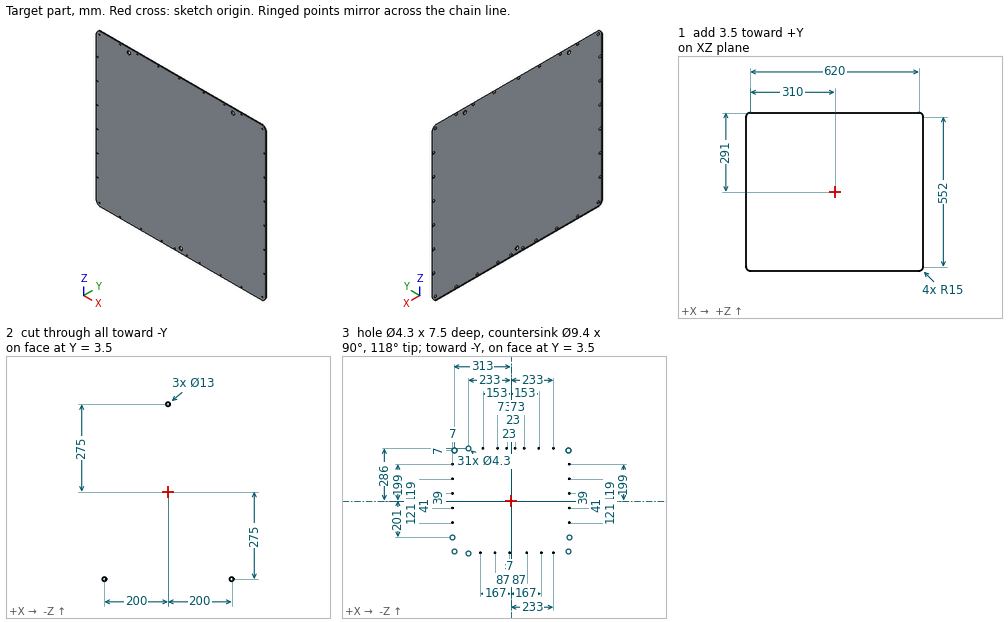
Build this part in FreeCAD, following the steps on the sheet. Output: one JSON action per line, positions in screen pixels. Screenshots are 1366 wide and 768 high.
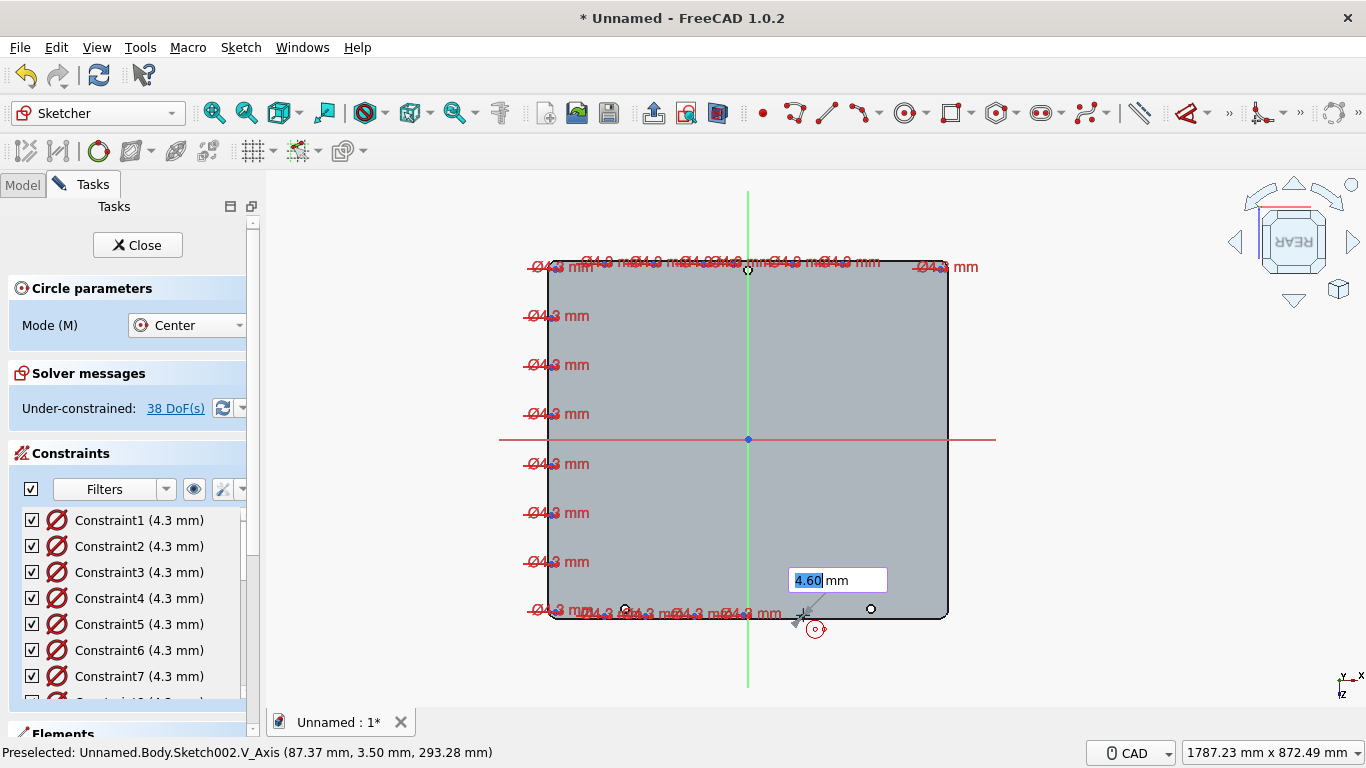
{"action": "type", "text": "4.3"}
{"action": "key", "text": "Return"}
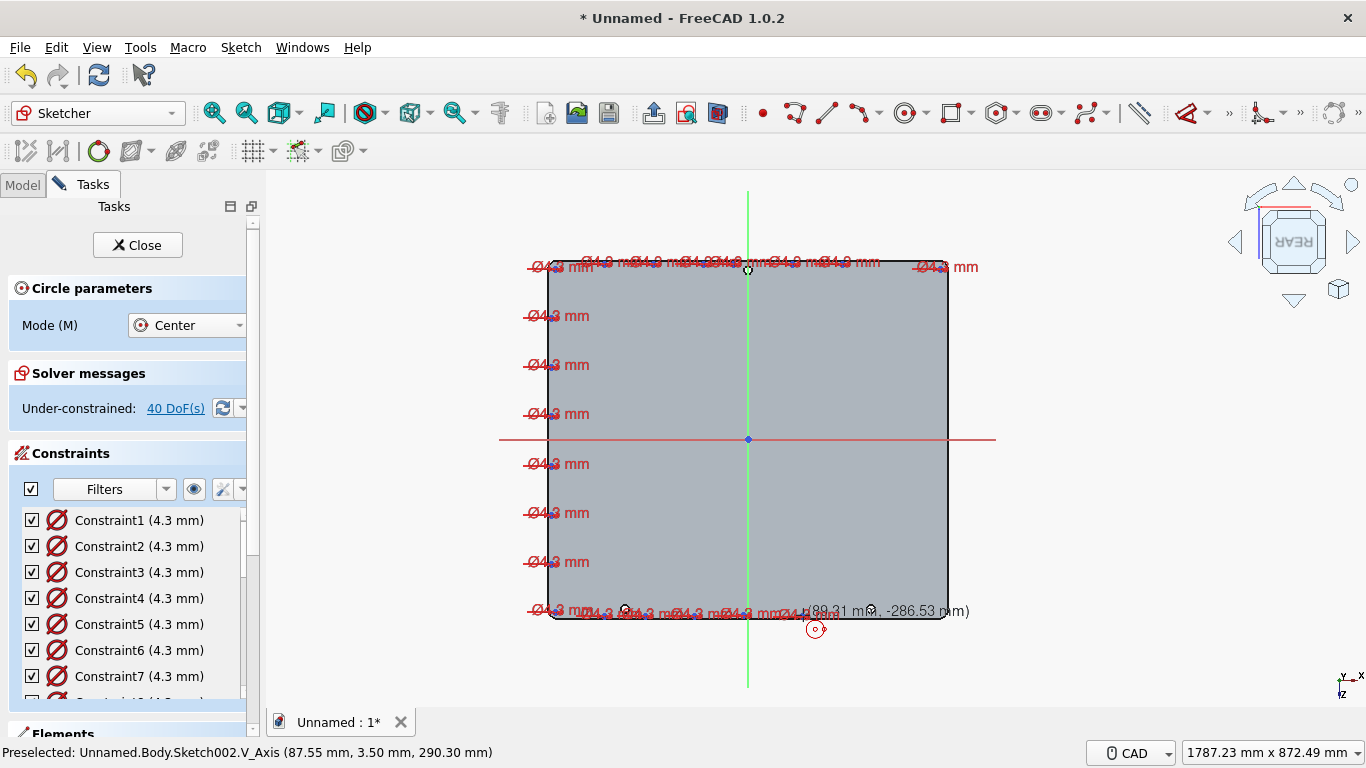
{"action": "scroll", "coordinate": [851, 616], "scroll_direction": "up", "scroll_amount": 15}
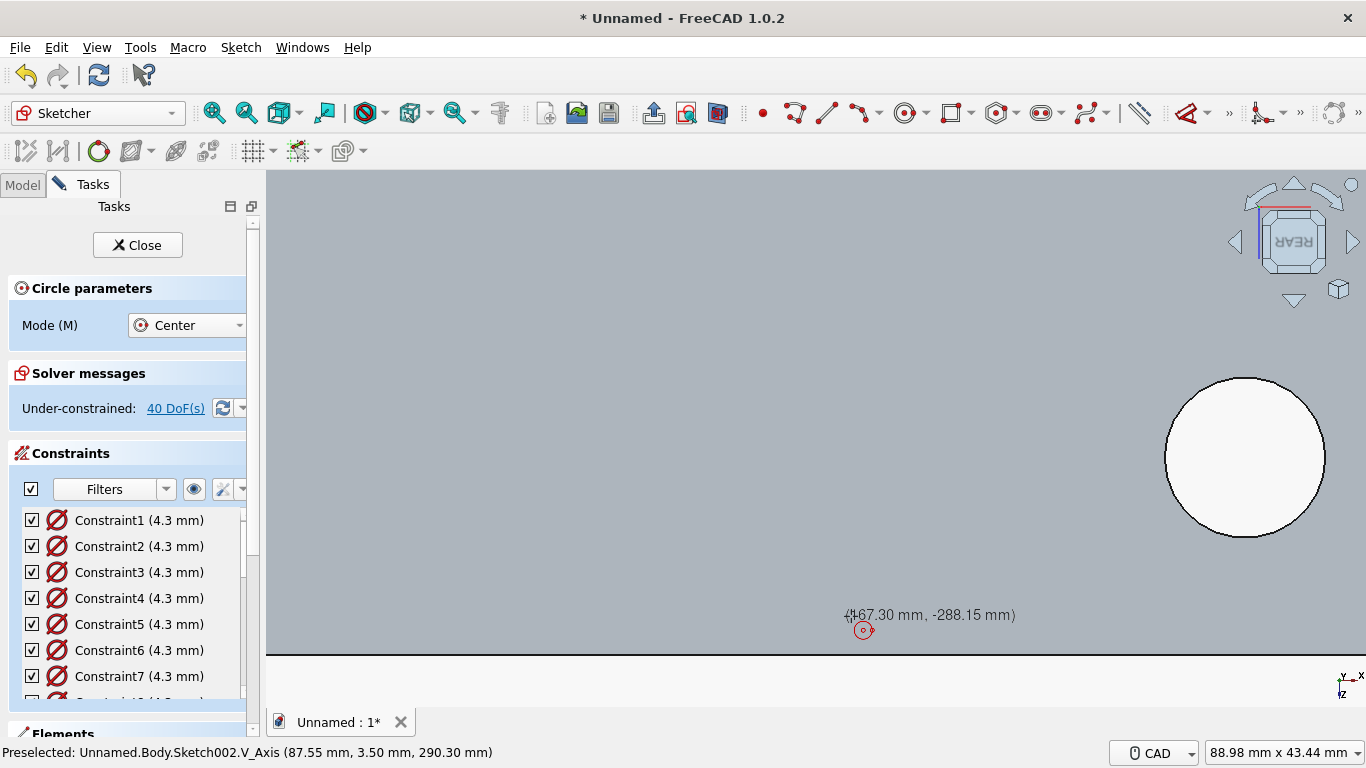
{"action": "scroll", "coordinate": [851, 616], "scroll_direction": "down", "scroll_amount": 15}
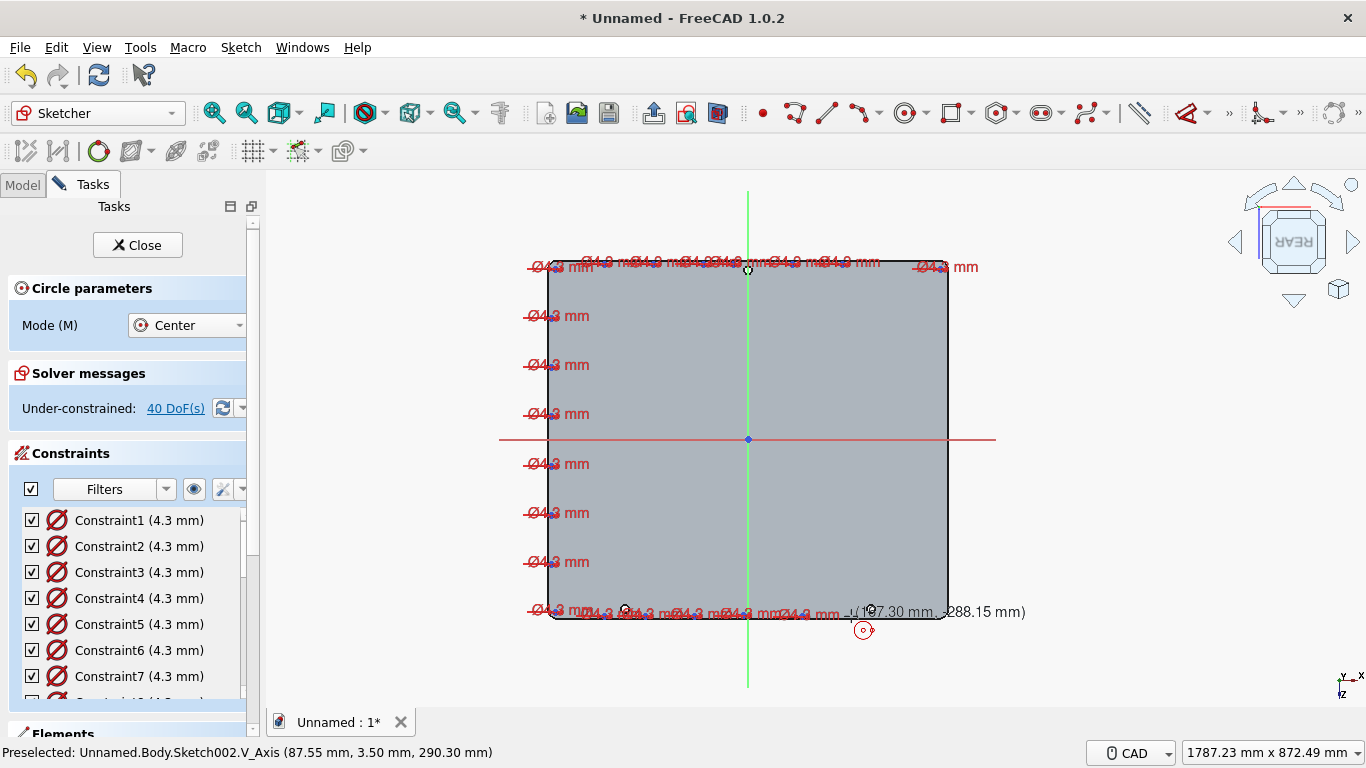
{"action": "left_click", "coordinate": [851, 616]}
{"action": "mouse_move", "coordinate": [852, 615]}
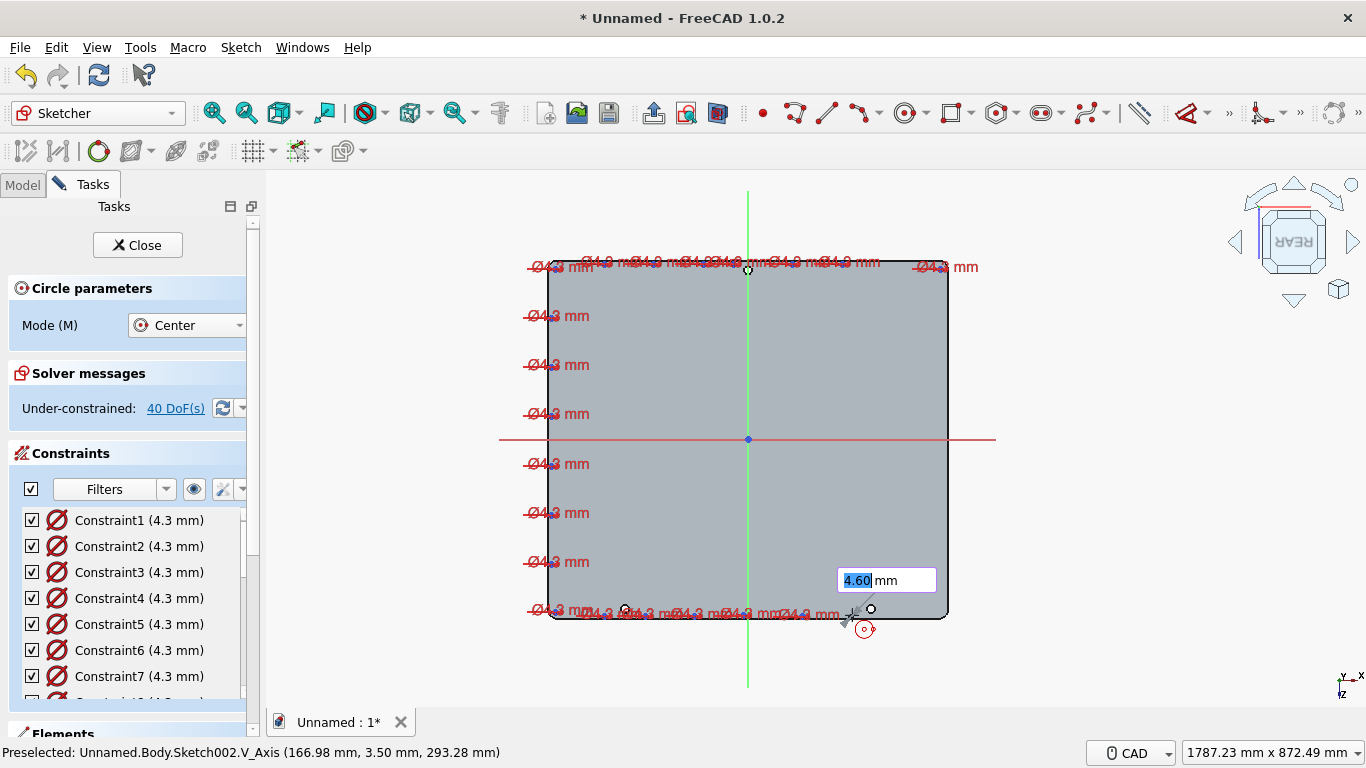
{"action": "type", "text": "4.3"}
{"action": "key", "text": "Return"}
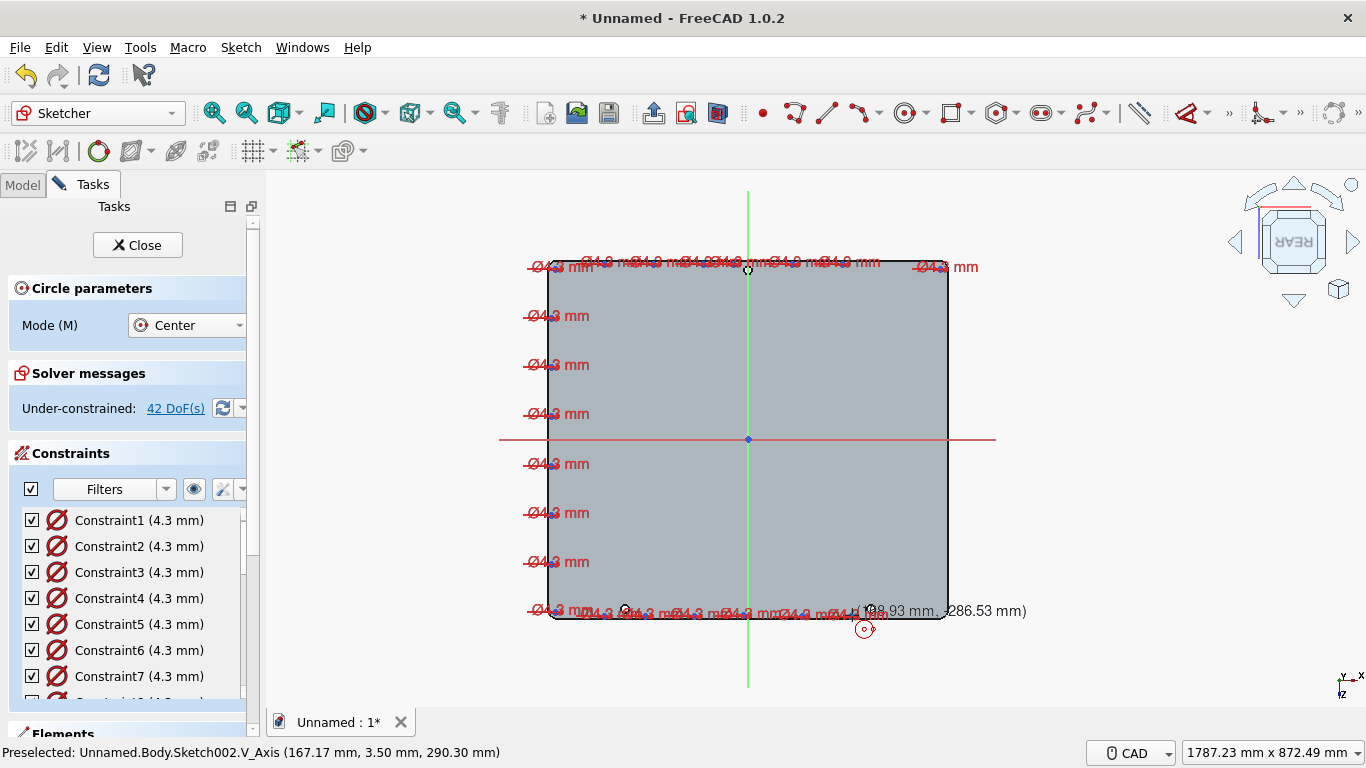
{"action": "scroll", "coordinate": [941, 611], "scroll_direction": "up", "scroll_amount": 15}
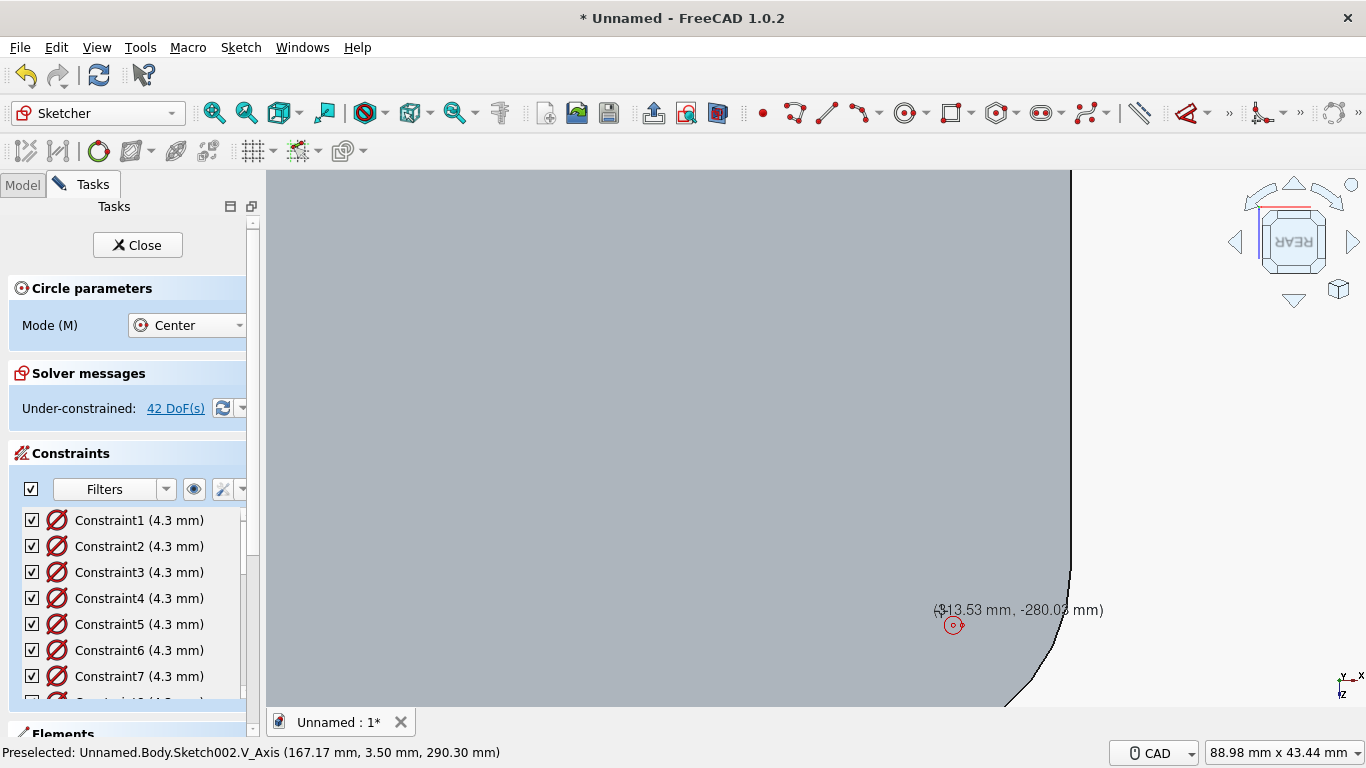
{"action": "scroll", "coordinate": [941, 611], "scroll_direction": "down", "scroll_amount": 15}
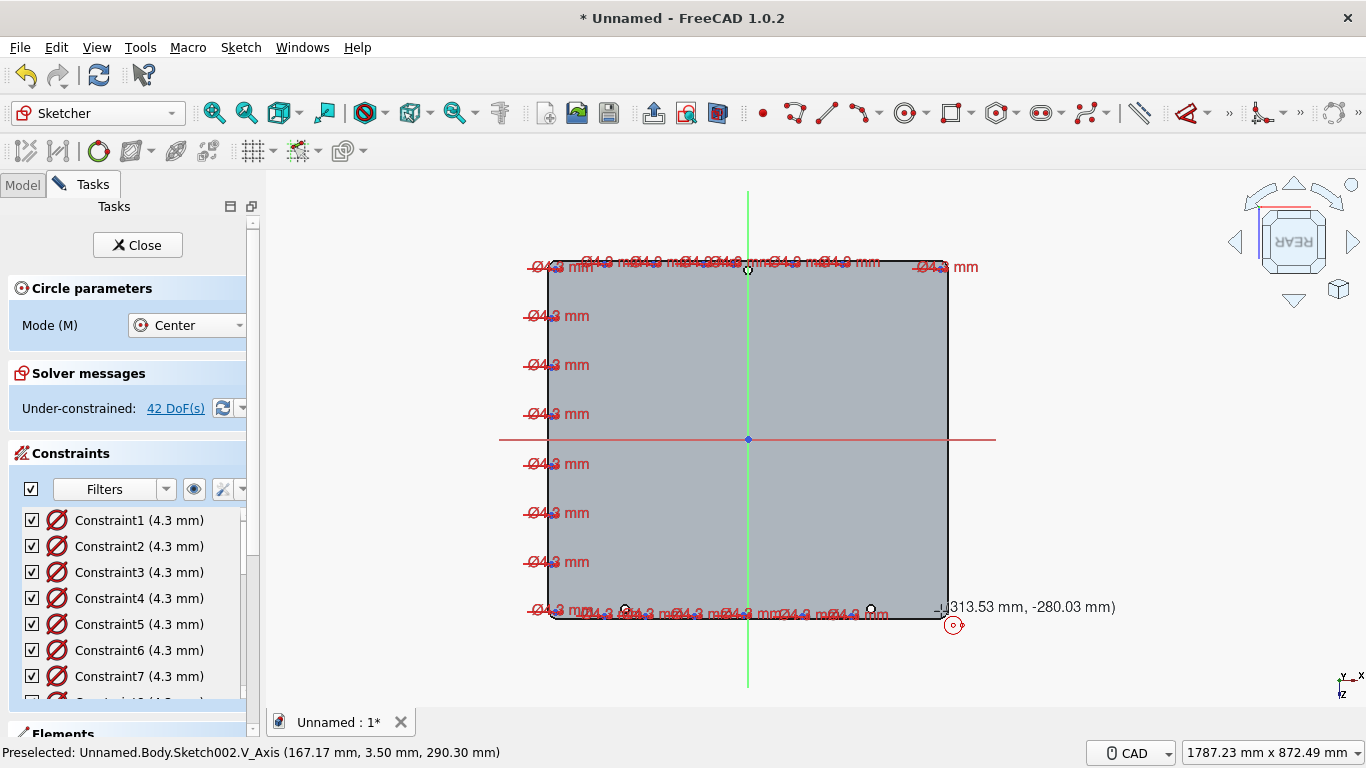
{"action": "left_click", "coordinate": [941, 611]}
{"action": "mouse_move", "coordinate": [942, 610]}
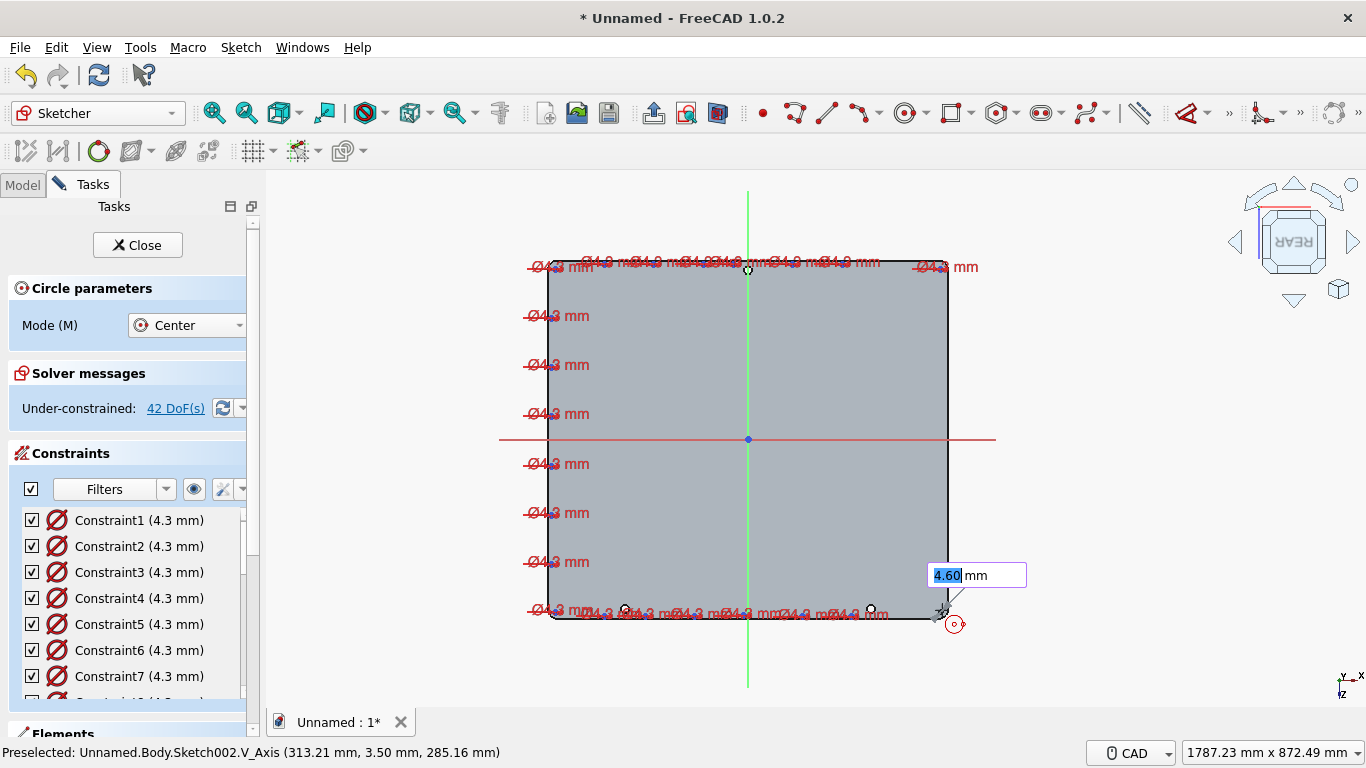
{"action": "type", "text": "4.3"}
{"action": "key", "text": "Return"}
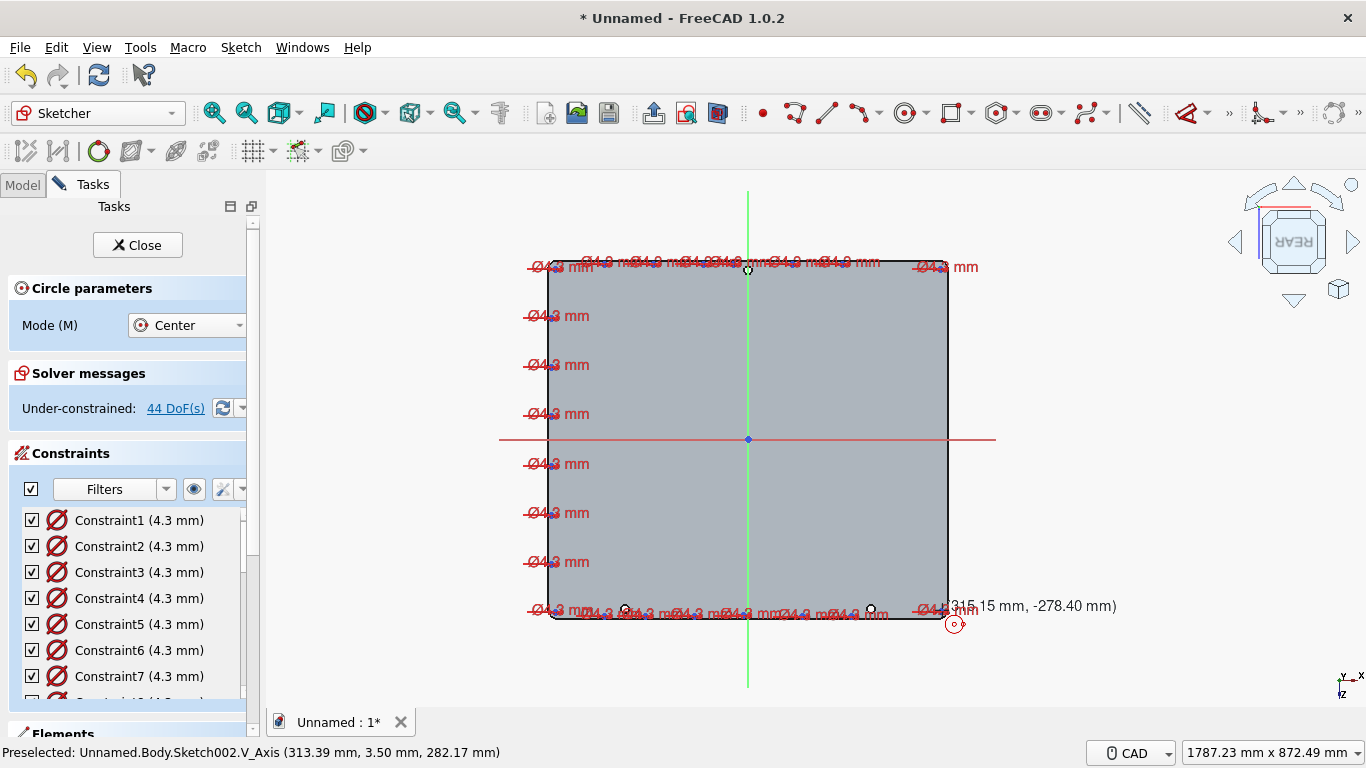
{"action": "scroll", "coordinate": [945, 563], "scroll_direction": "up", "scroll_amount": 15}